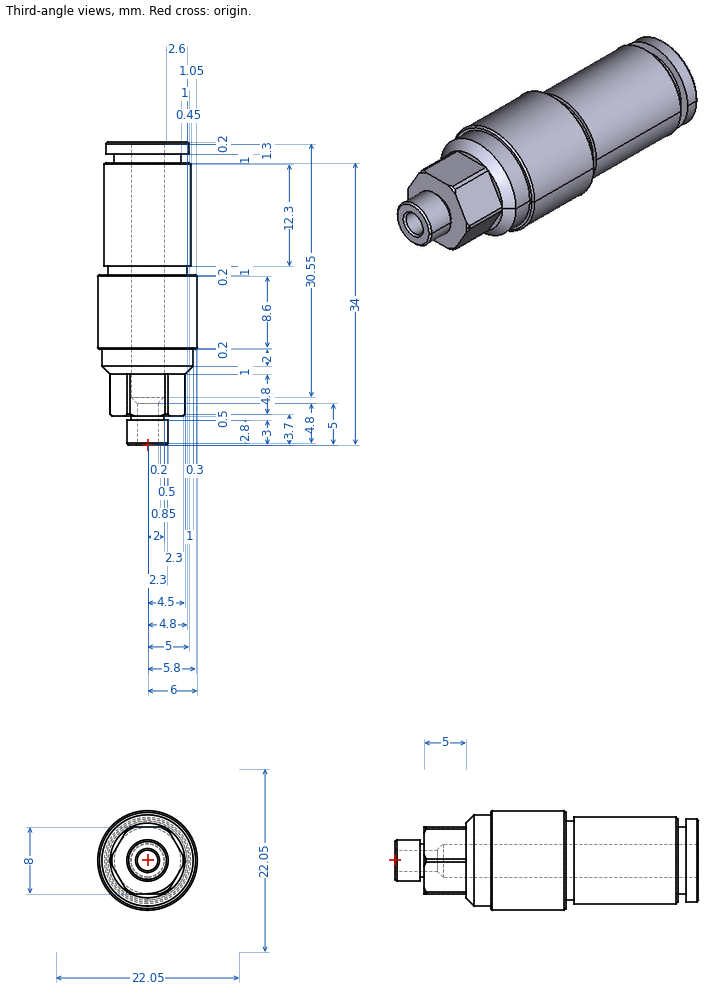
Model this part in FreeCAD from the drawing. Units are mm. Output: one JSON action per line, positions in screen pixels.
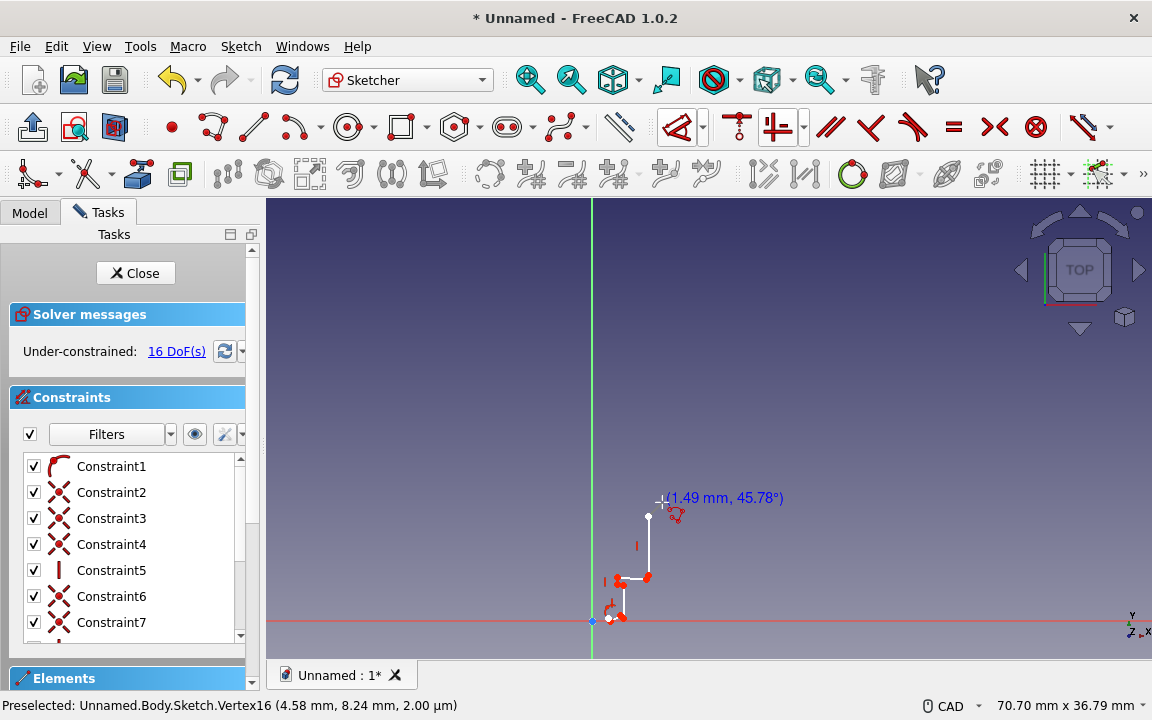
{"action": "left_click", "coordinate": [661, 502]}
{"action": "left_click", "coordinate": [661, 477]}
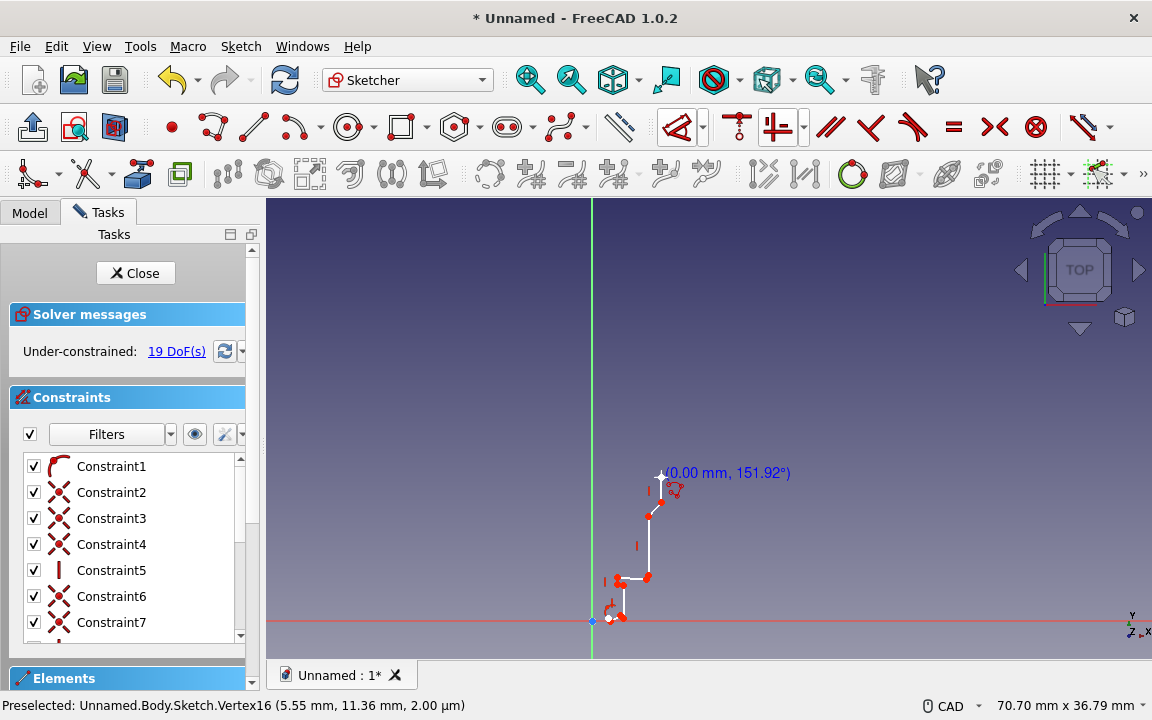
{"action": "scroll", "coordinate": [665, 477], "scroll_direction": "up", "scroll_amount": 8}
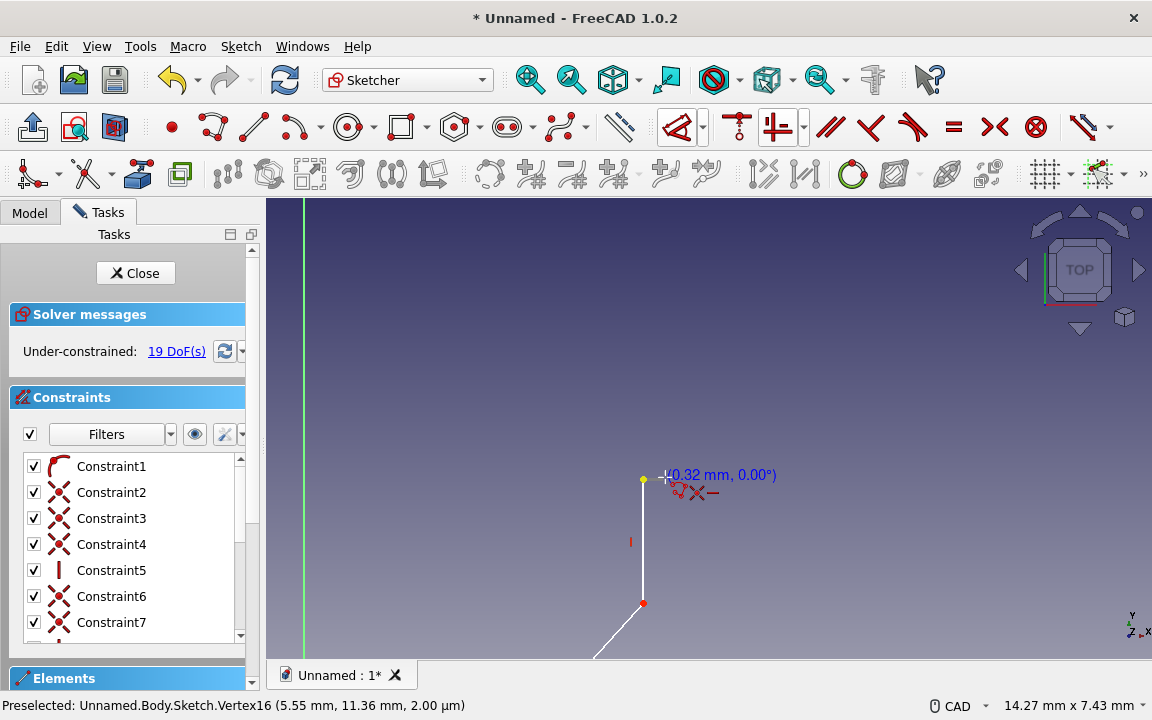
{"action": "left_click", "coordinate": [664, 475]}
{"action": "left_click", "coordinate": [676, 463]}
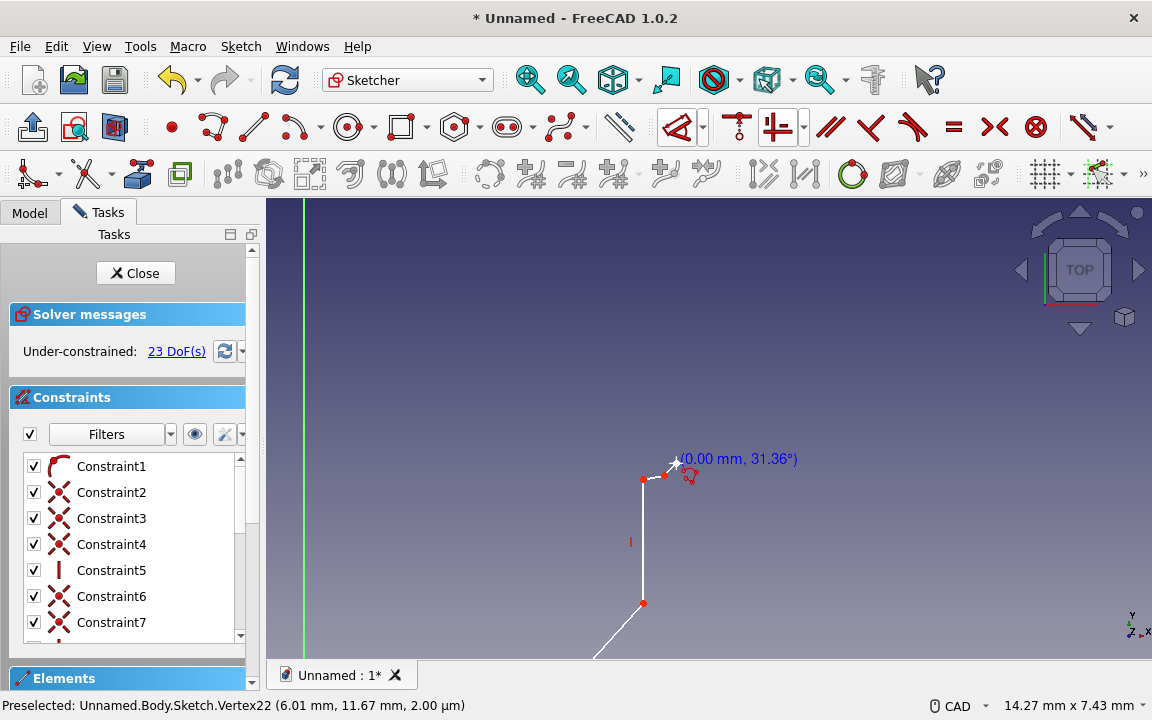
{"action": "scroll", "coordinate": [664, 487], "scroll_direction": "down", "scroll_amount": 10}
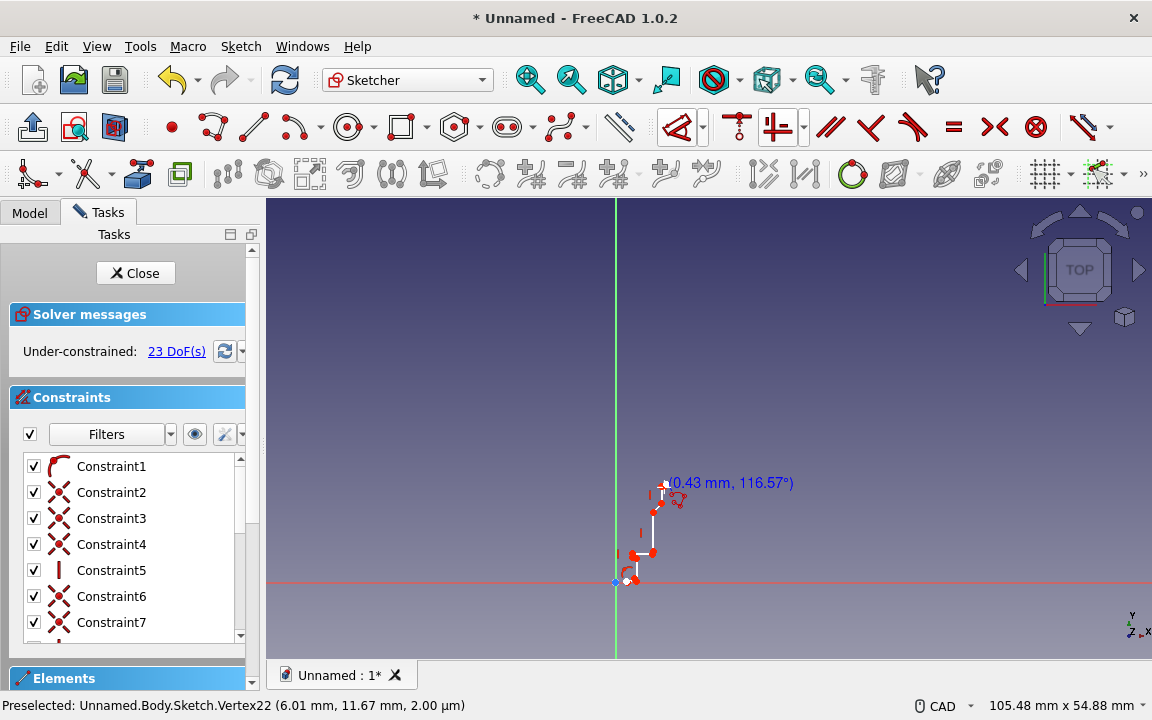
{"action": "left_click", "coordinate": [666, 412]}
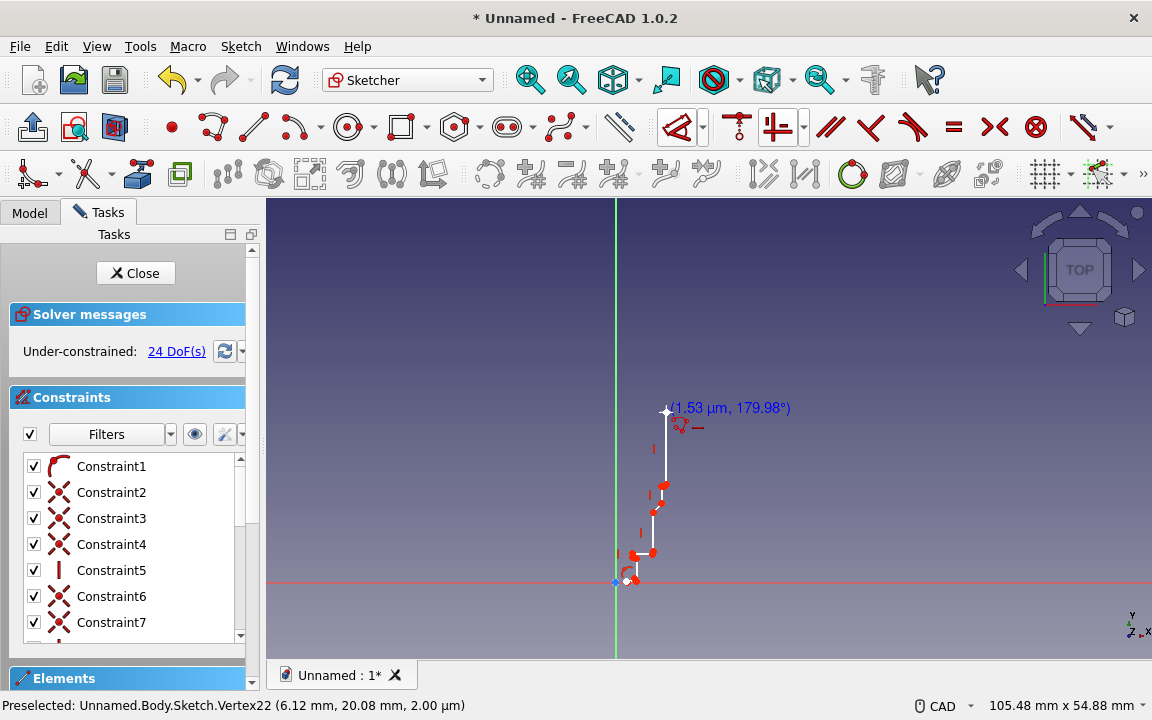
{"action": "scroll", "coordinate": [664, 410], "scroll_direction": "up", "scroll_amount": 10}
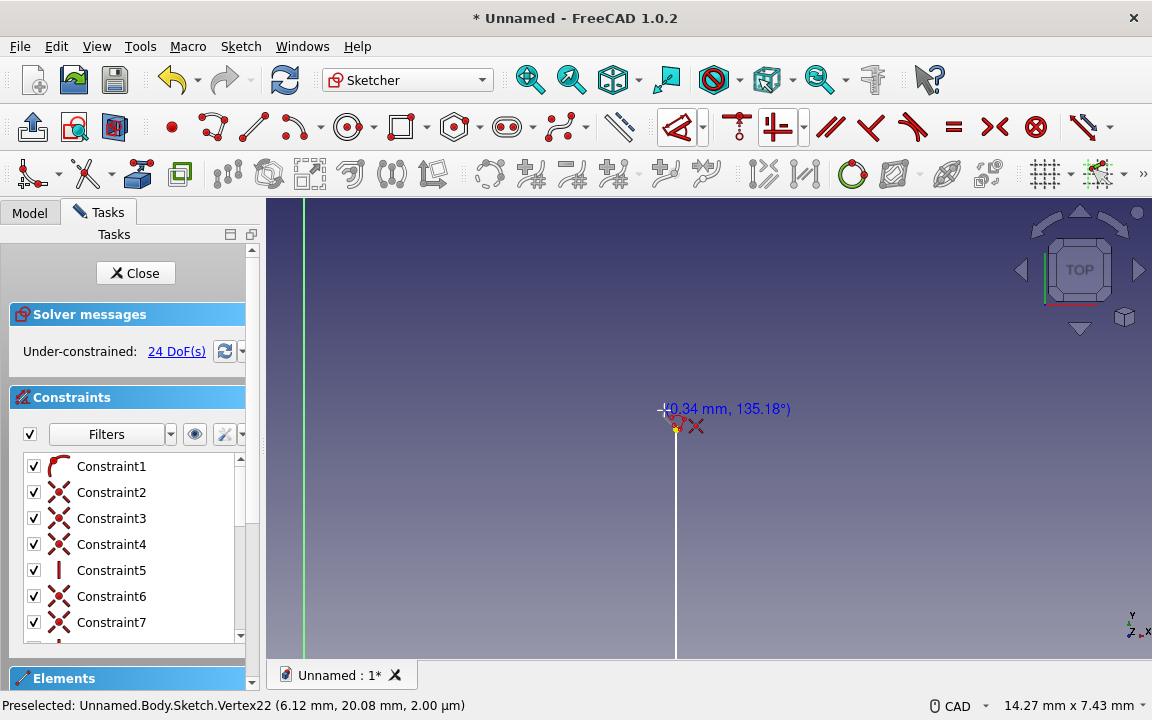
{"action": "left_click", "coordinate": [664, 410]}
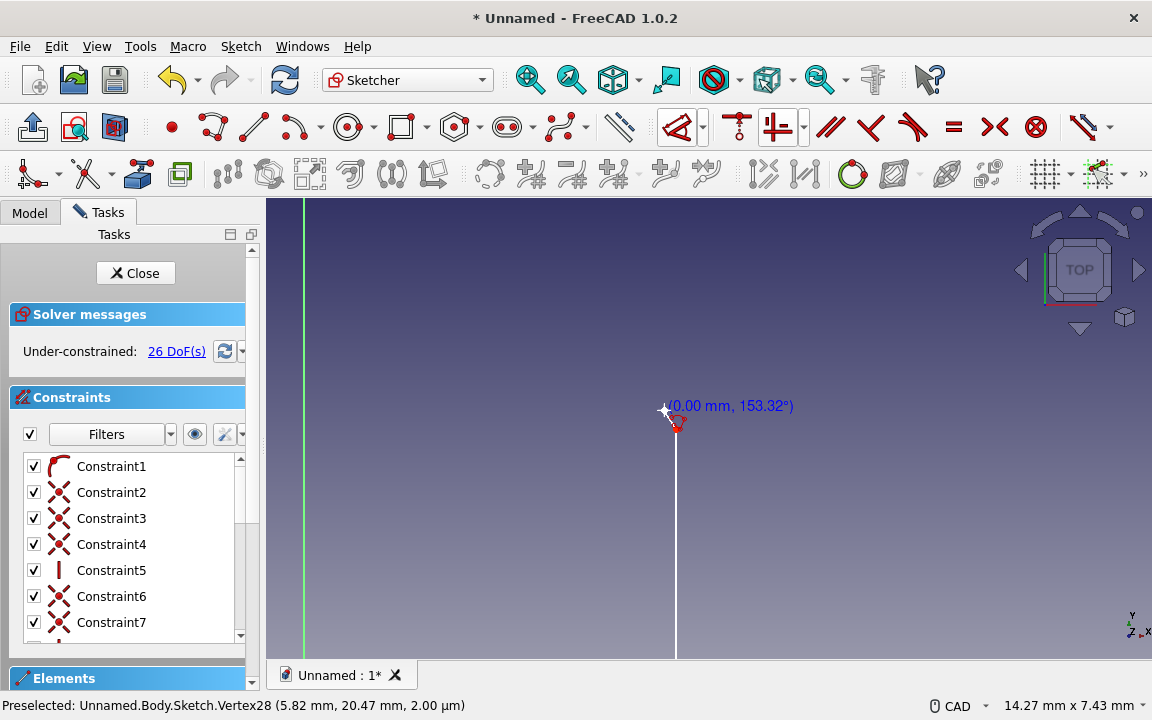
{"action": "scroll", "coordinate": [664, 409], "scroll_direction": "down", "scroll_amount": 10}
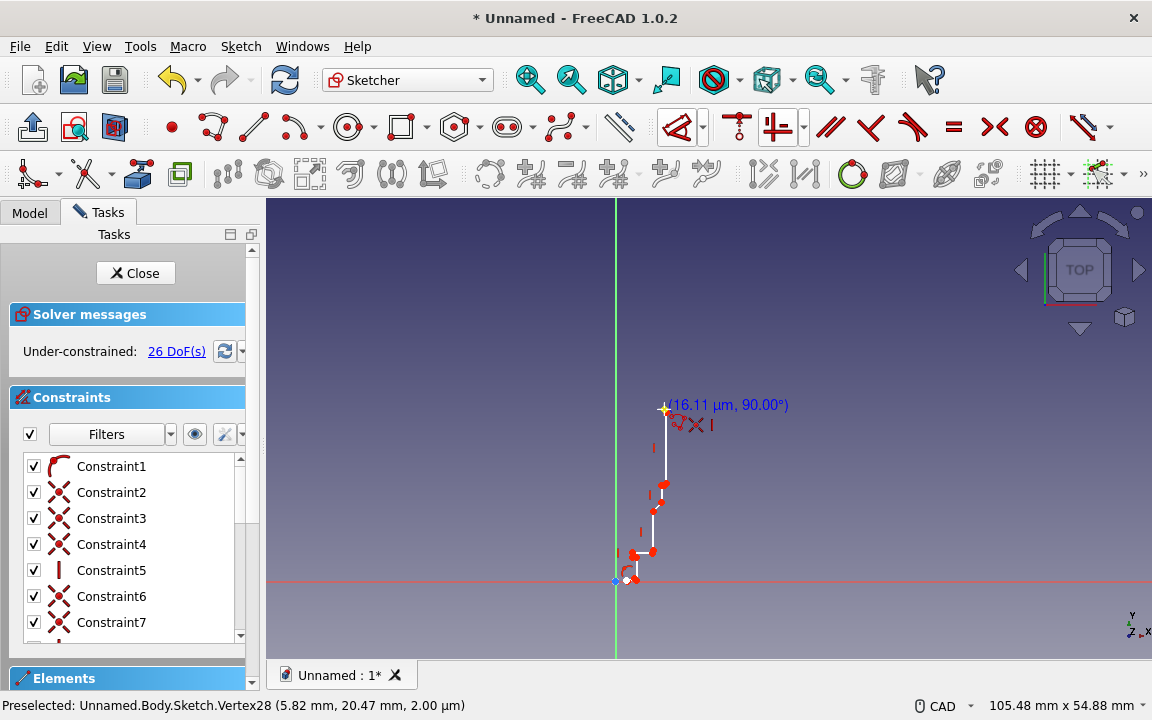
{"action": "scroll", "coordinate": [656, 410], "scroll_direction": "up", "scroll_amount": 3}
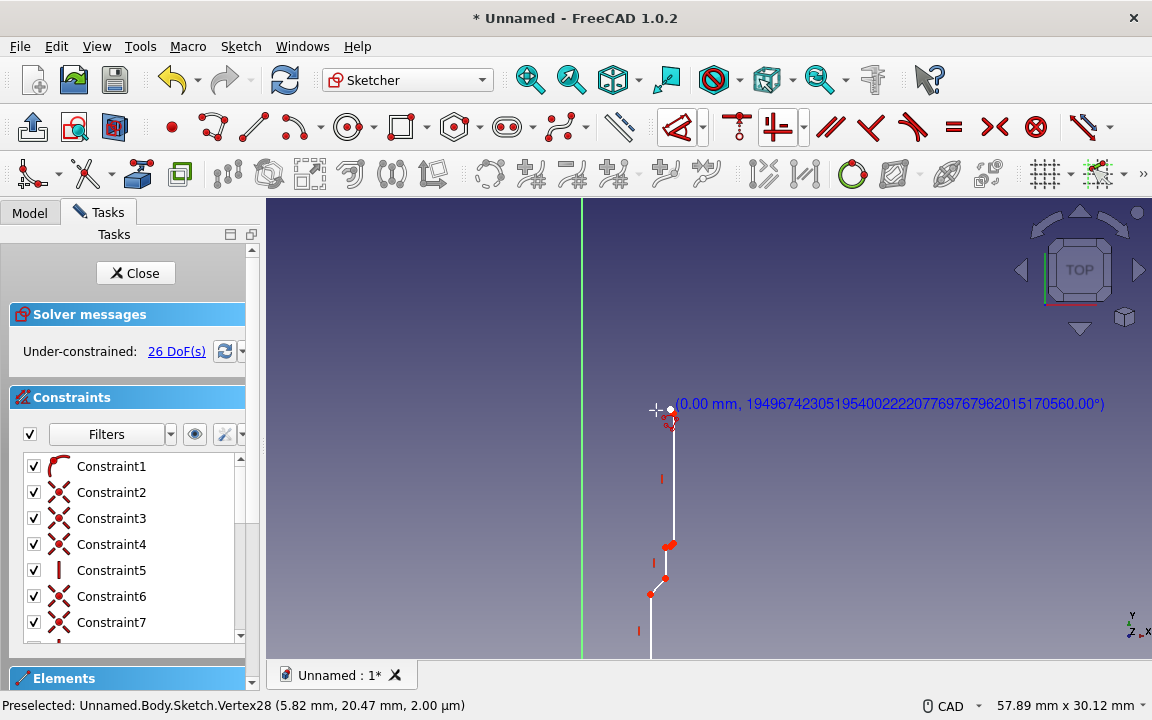
{"action": "left_click", "coordinate": [655, 409]}
{"action": "left_click", "coordinate": [655, 394]}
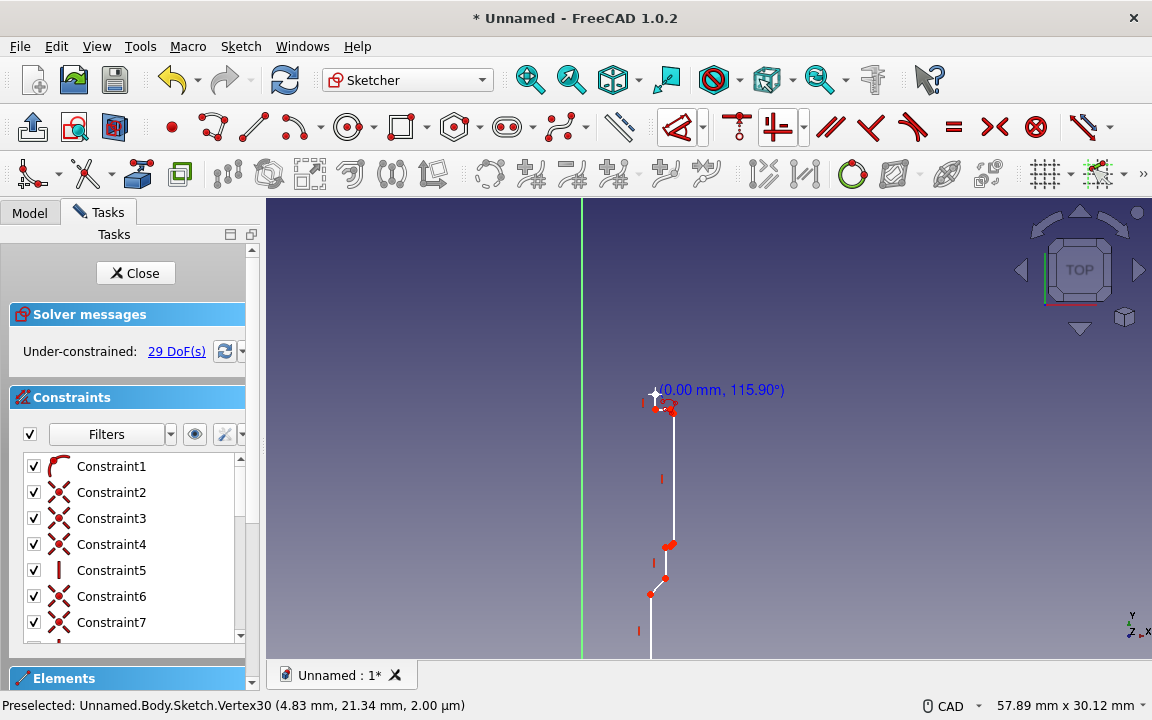
{"action": "scroll", "coordinate": [662, 394], "scroll_direction": "up", "scroll_amount": 5}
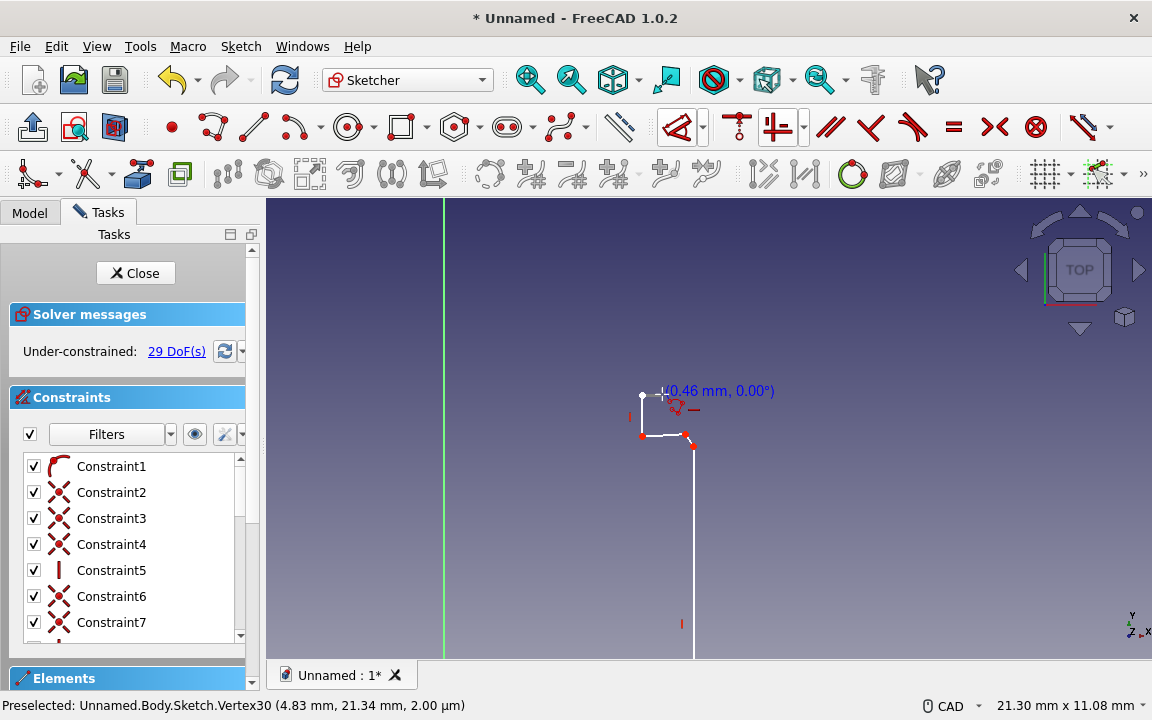
{"action": "left_click", "coordinate": [660, 393]}